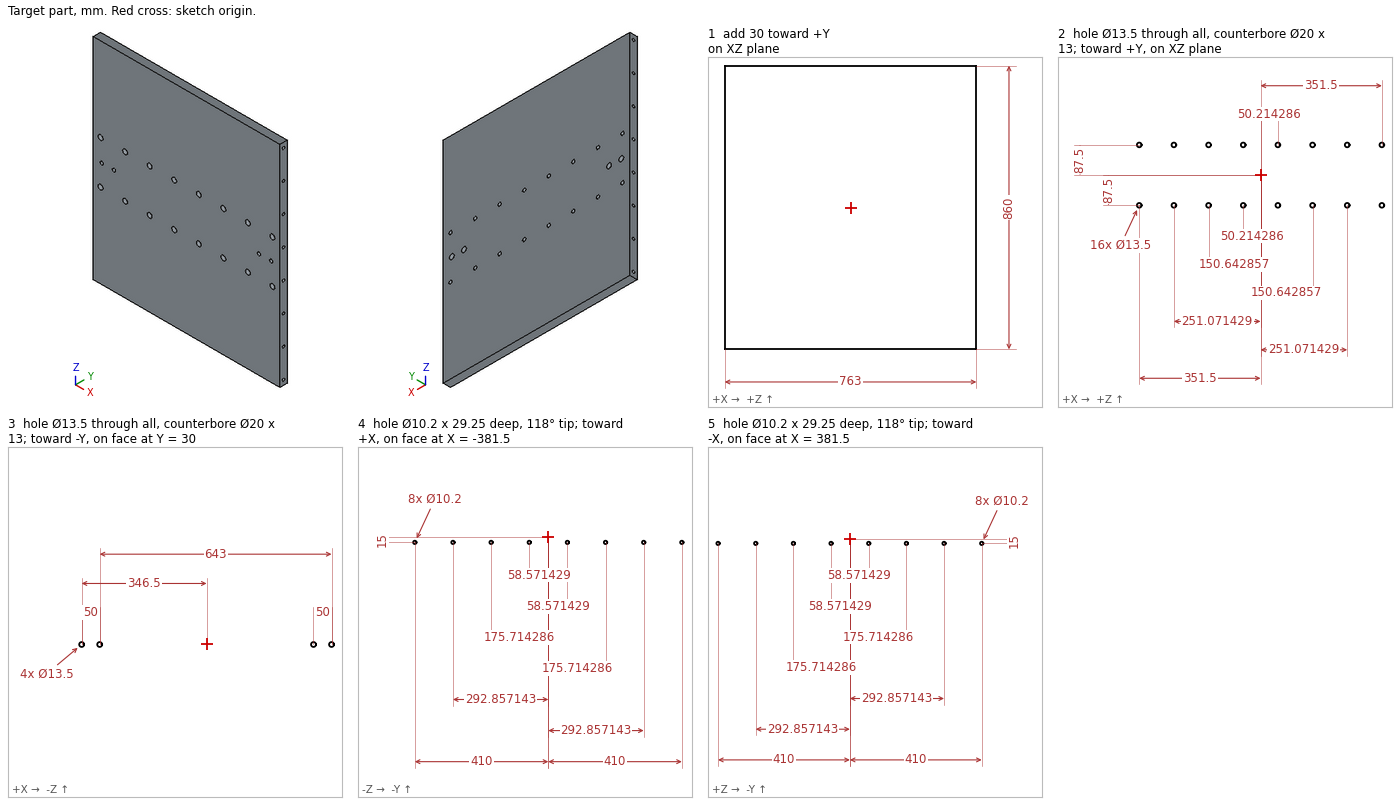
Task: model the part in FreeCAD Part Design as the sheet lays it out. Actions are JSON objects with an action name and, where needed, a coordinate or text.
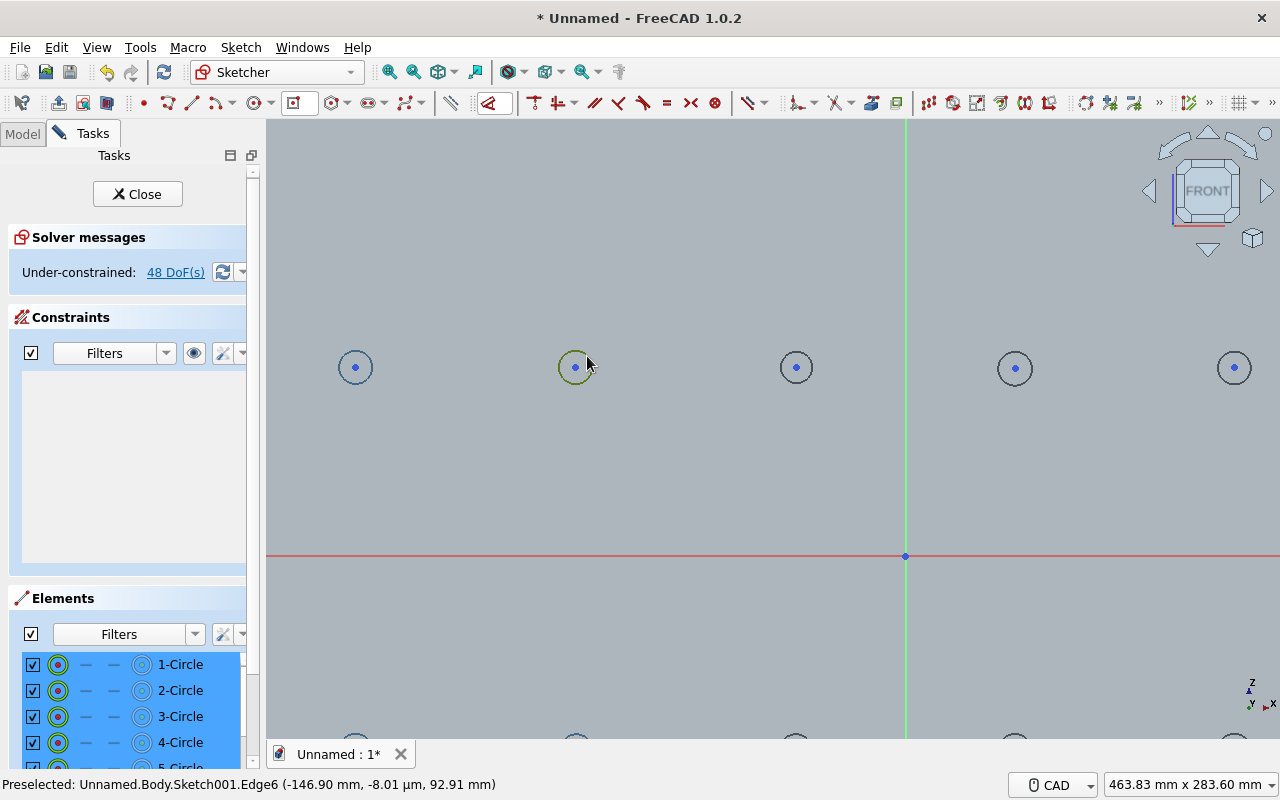
{"action": "scroll", "coordinate": [587, 355], "scroll_direction": "down", "scroll_amount": 5}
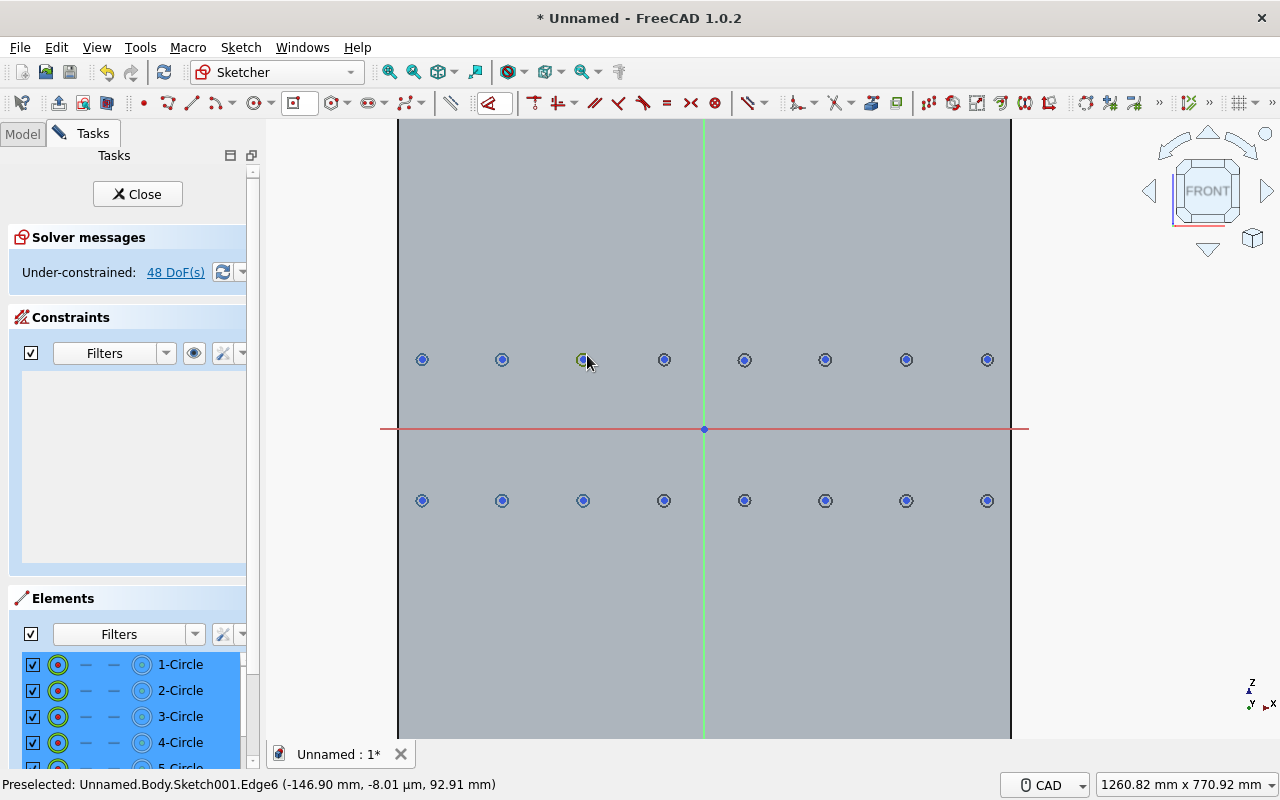
{"action": "scroll", "coordinate": [668, 497], "scroll_direction": "up", "scroll_amount": 5}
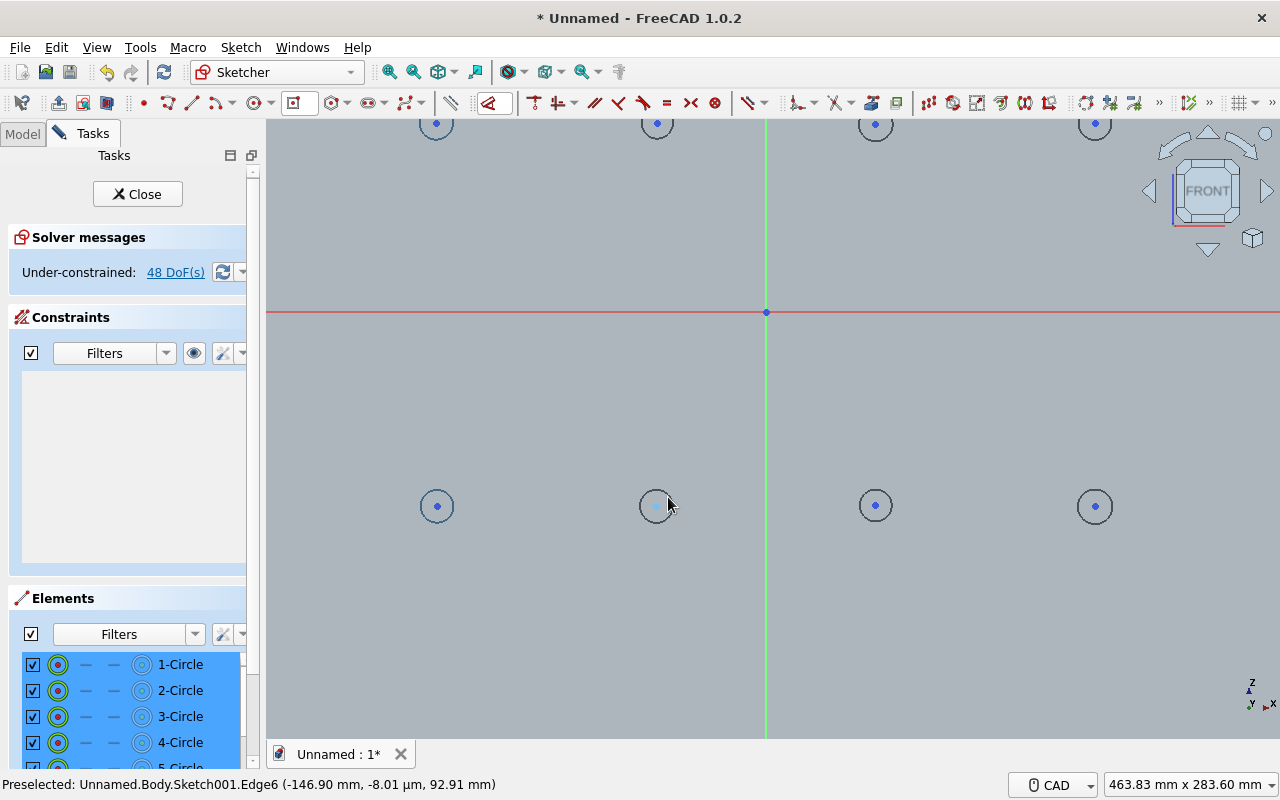
{"action": "left_click", "coordinate": [668, 495]}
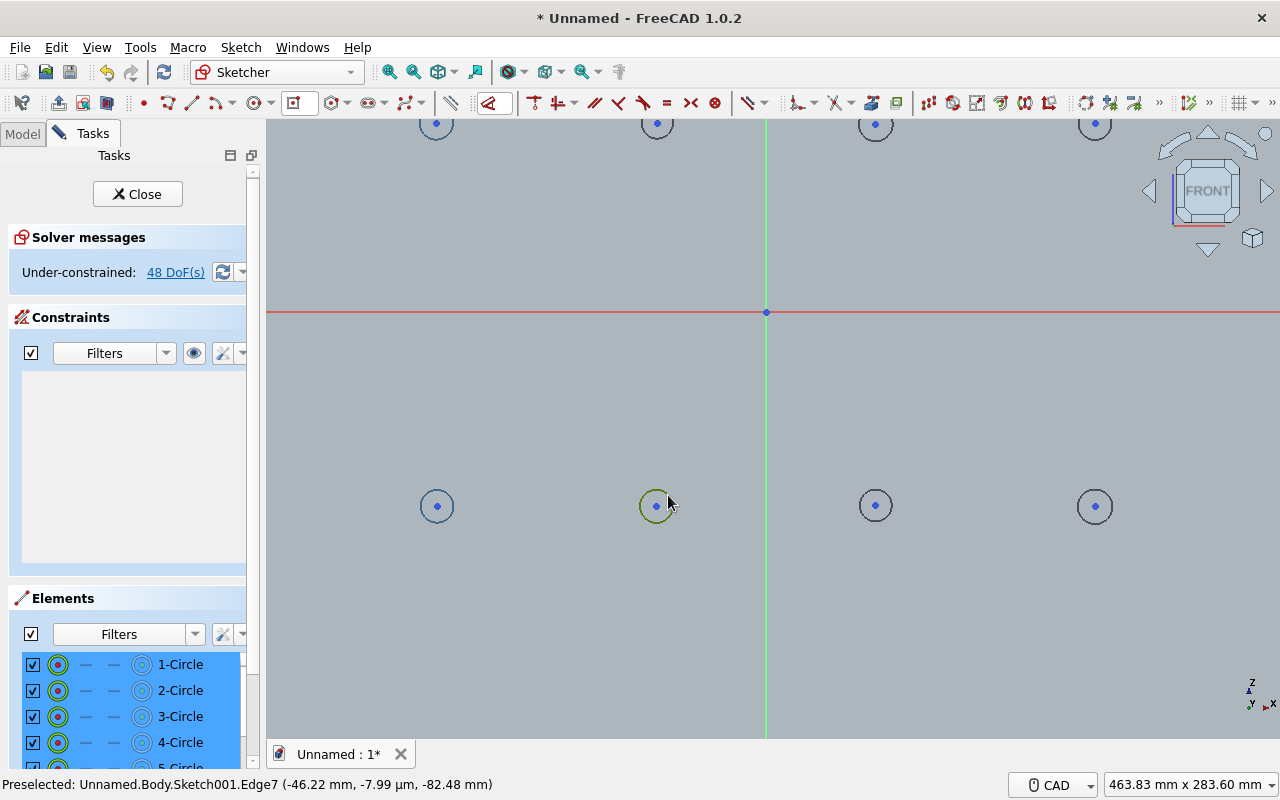
{"action": "scroll", "coordinate": [669, 497], "scroll_direction": "down", "scroll_amount": 5}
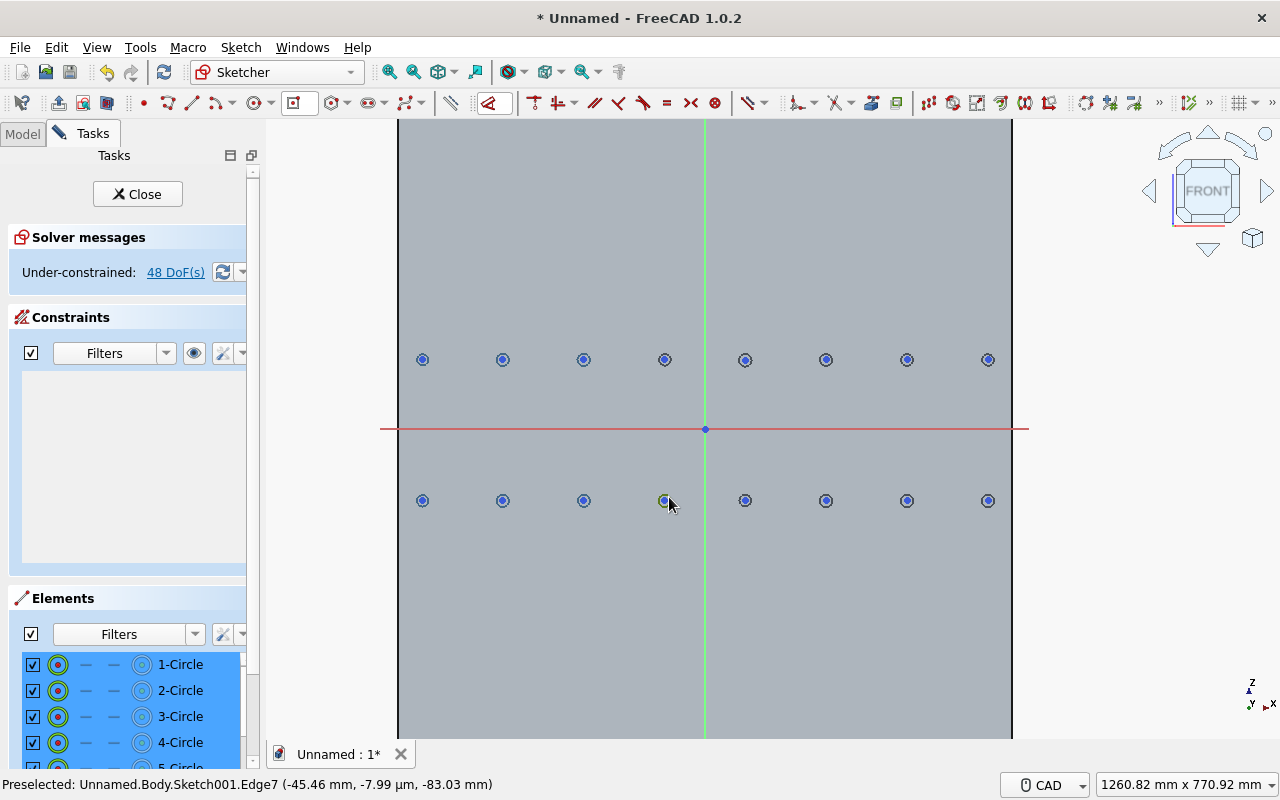
{"action": "scroll", "coordinate": [669, 356], "scroll_direction": "up", "scroll_amount": 5}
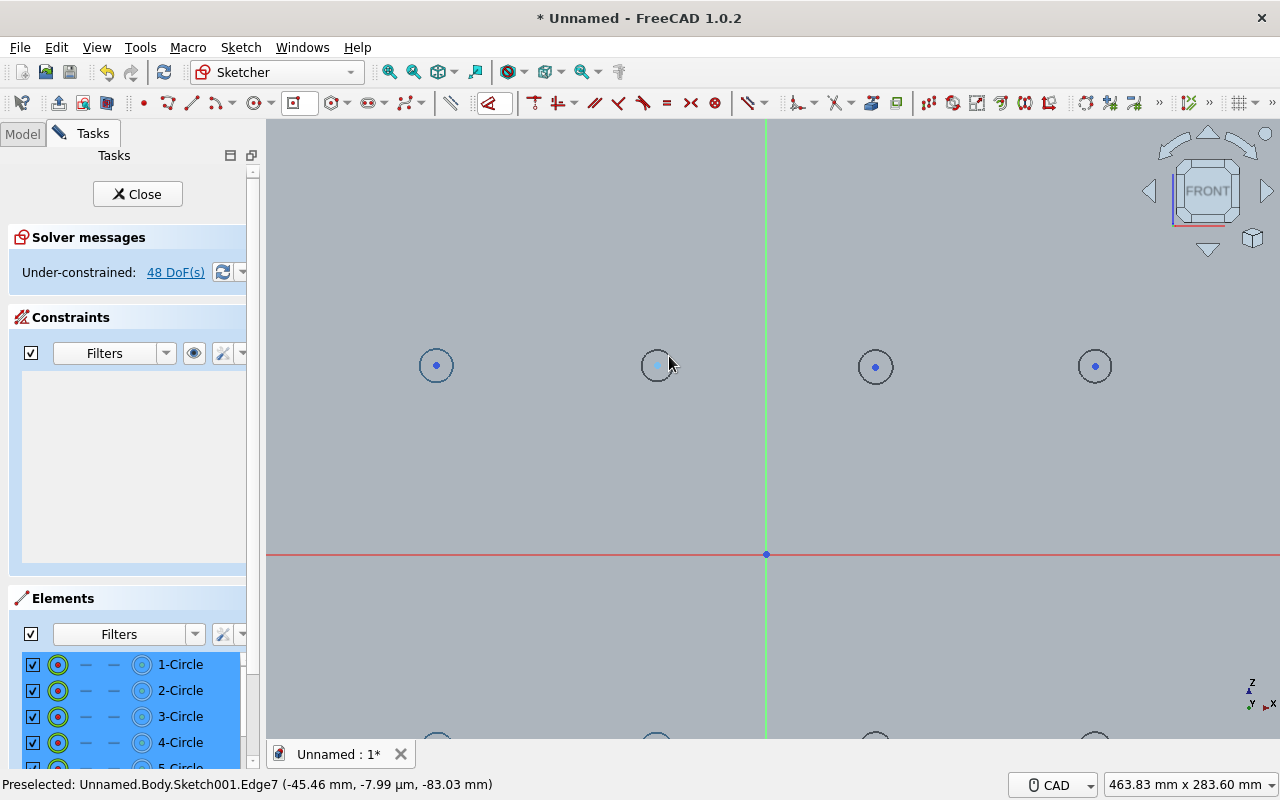
{"action": "left_click", "coordinate": [668, 355]}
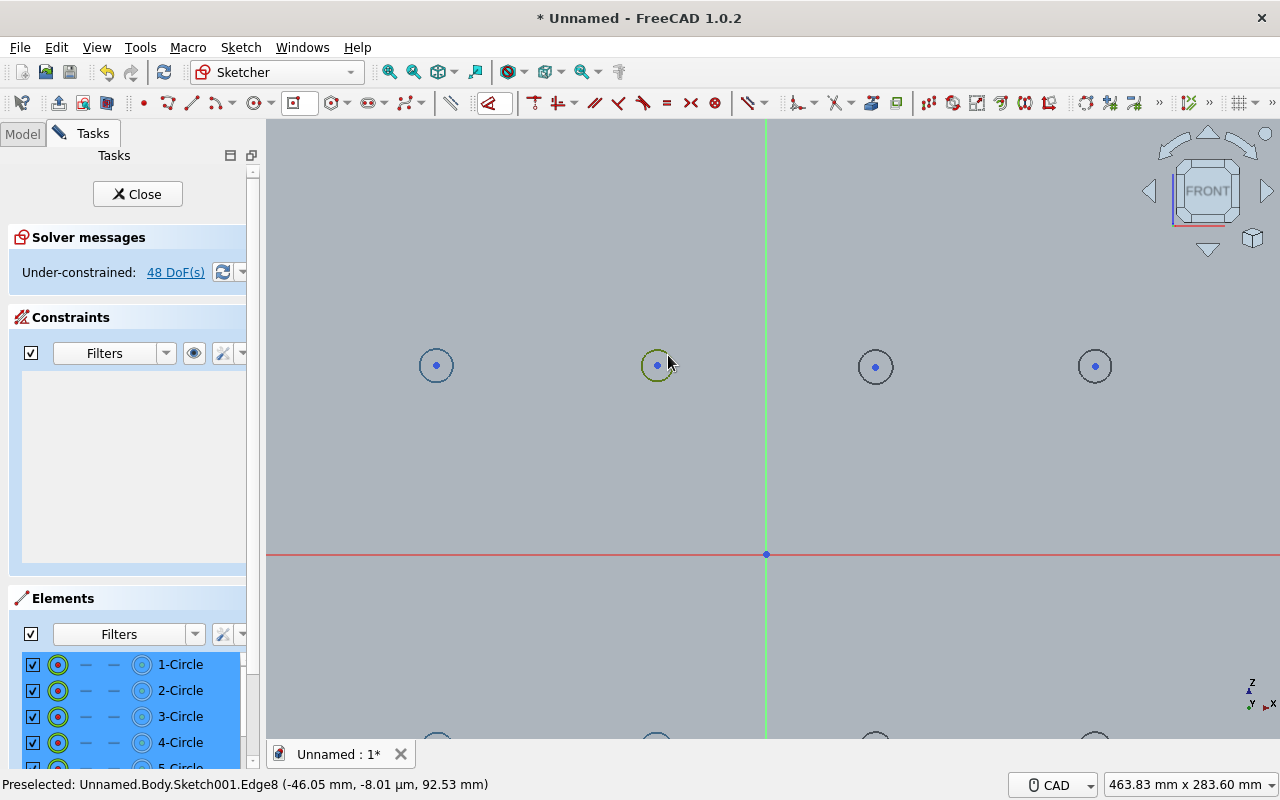
{"action": "left_click", "coordinate": [888, 355]}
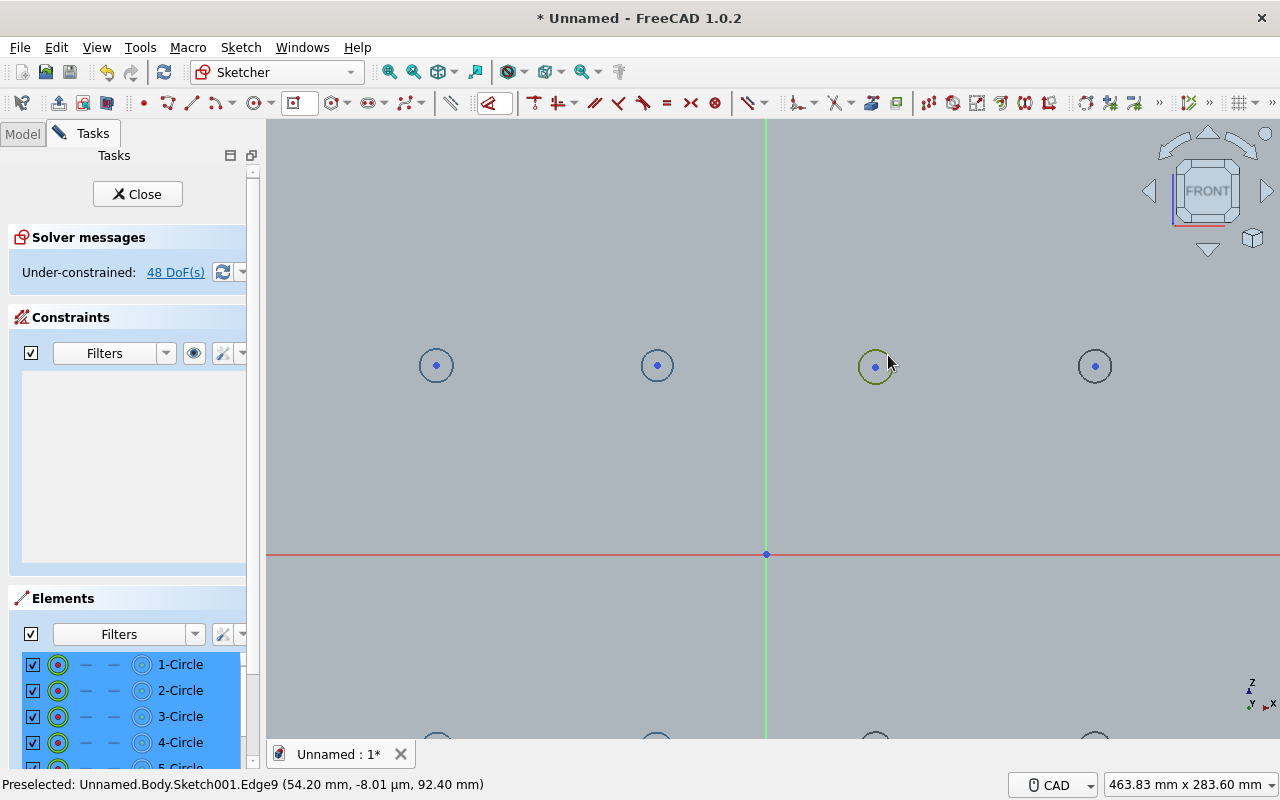
{"action": "scroll", "coordinate": [669, 356], "scroll_direction": "down", "scroll_amount": 5}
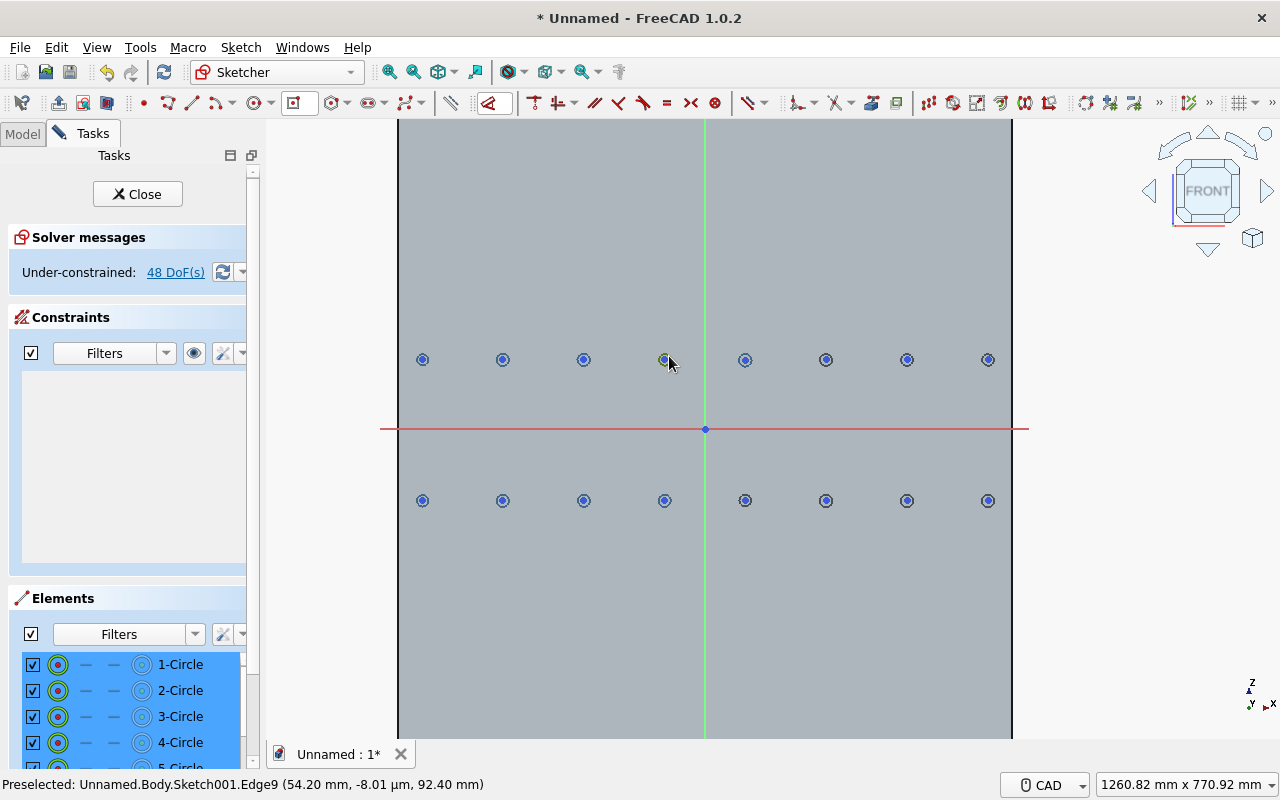
{"action": "scroll", "coordinate": [749, 496], "scroll_direction": "up", "scroll_amount": 5}